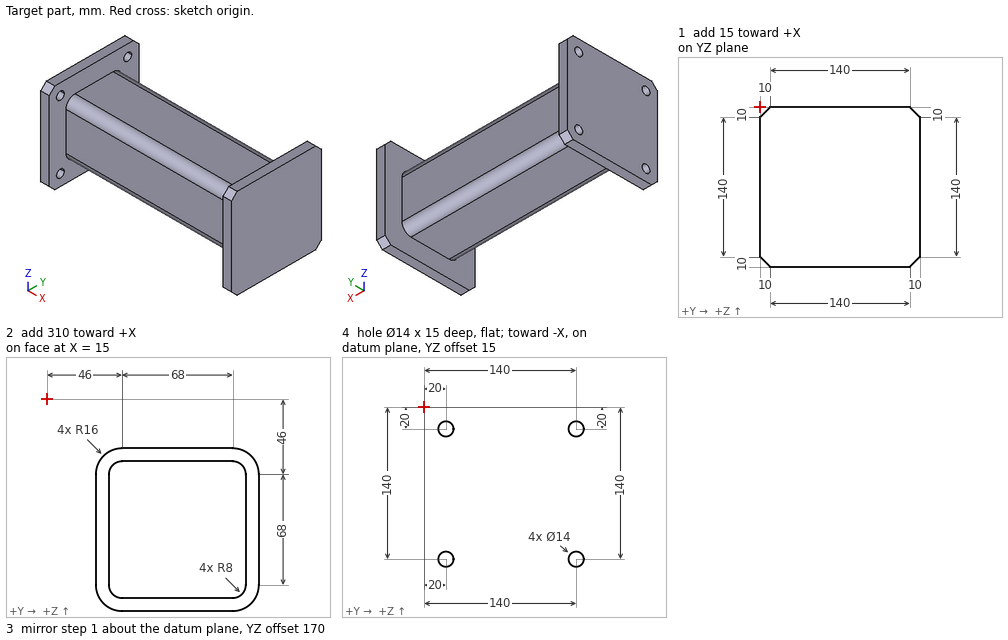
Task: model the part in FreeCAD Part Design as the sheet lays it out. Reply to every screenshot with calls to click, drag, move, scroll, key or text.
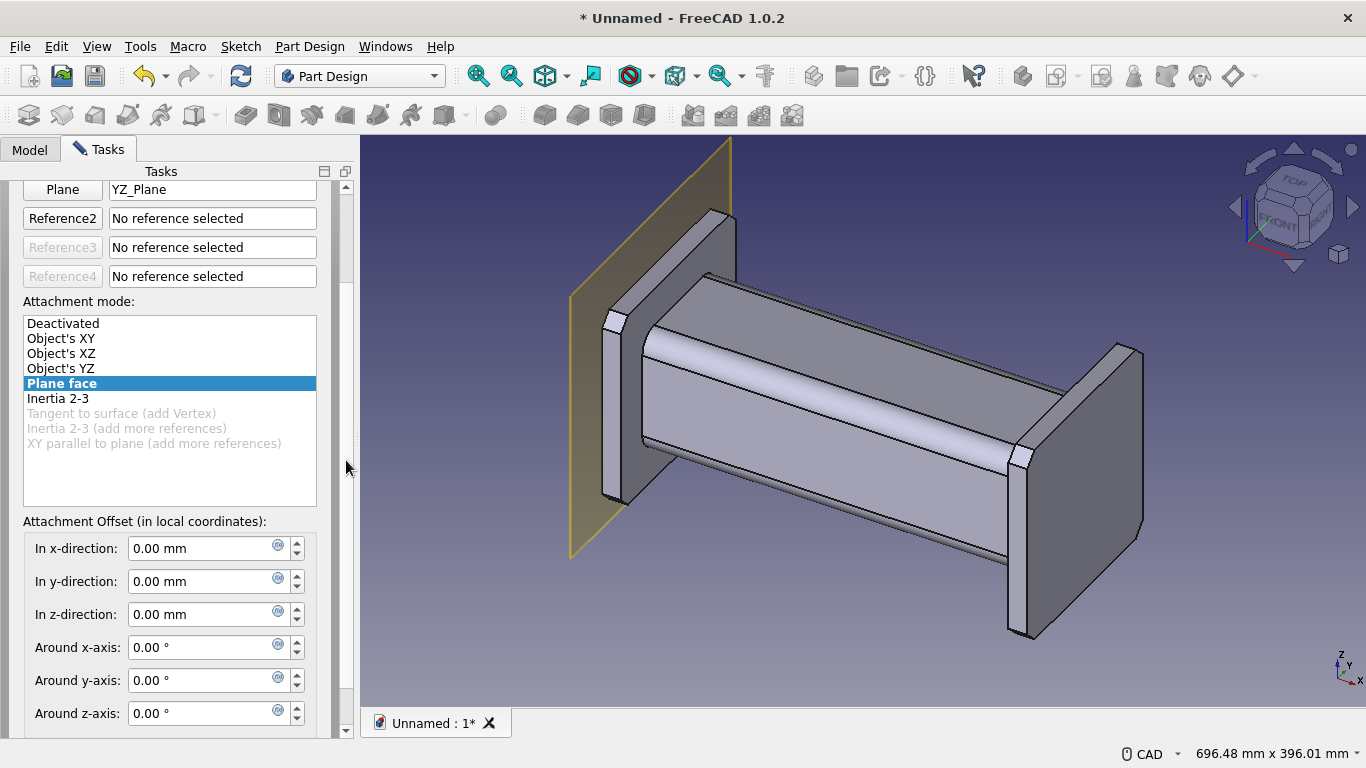
triple_click(210, 614)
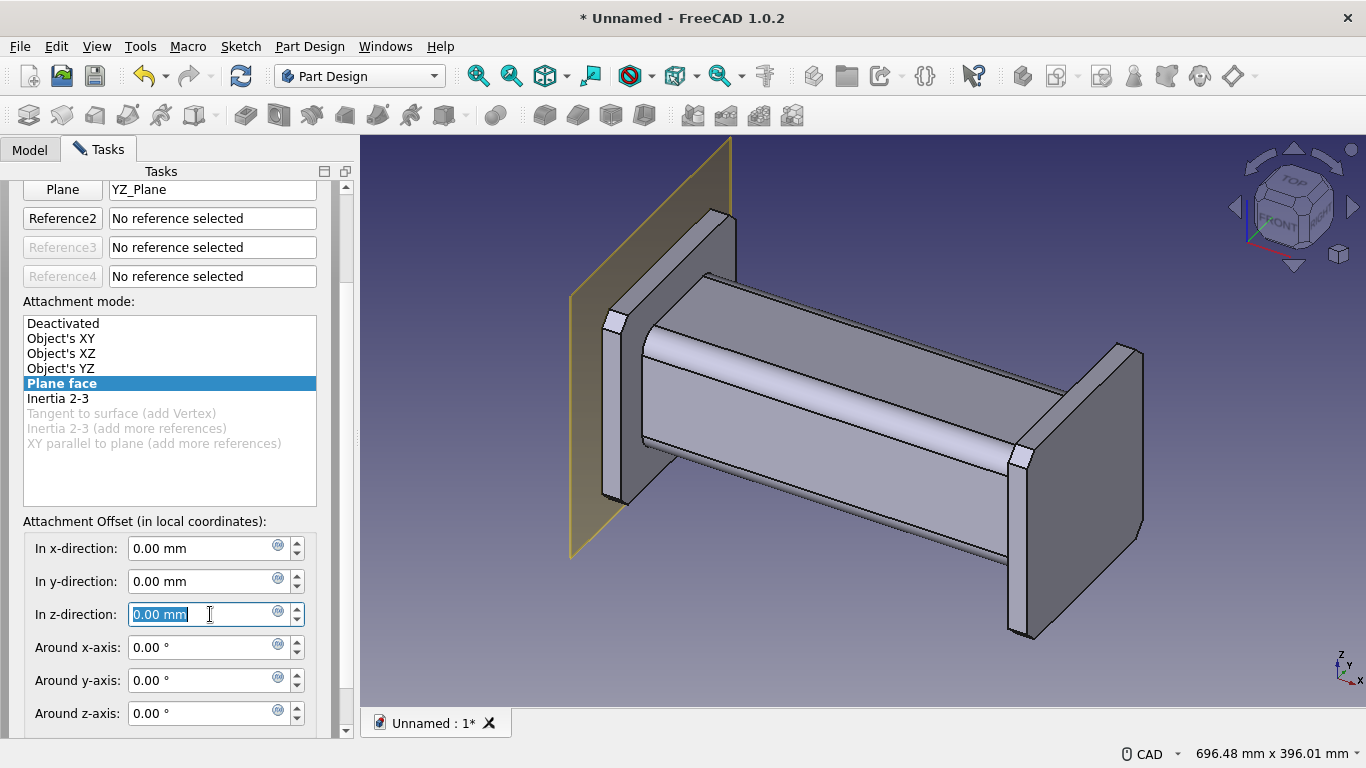
text(15)
key(Tab)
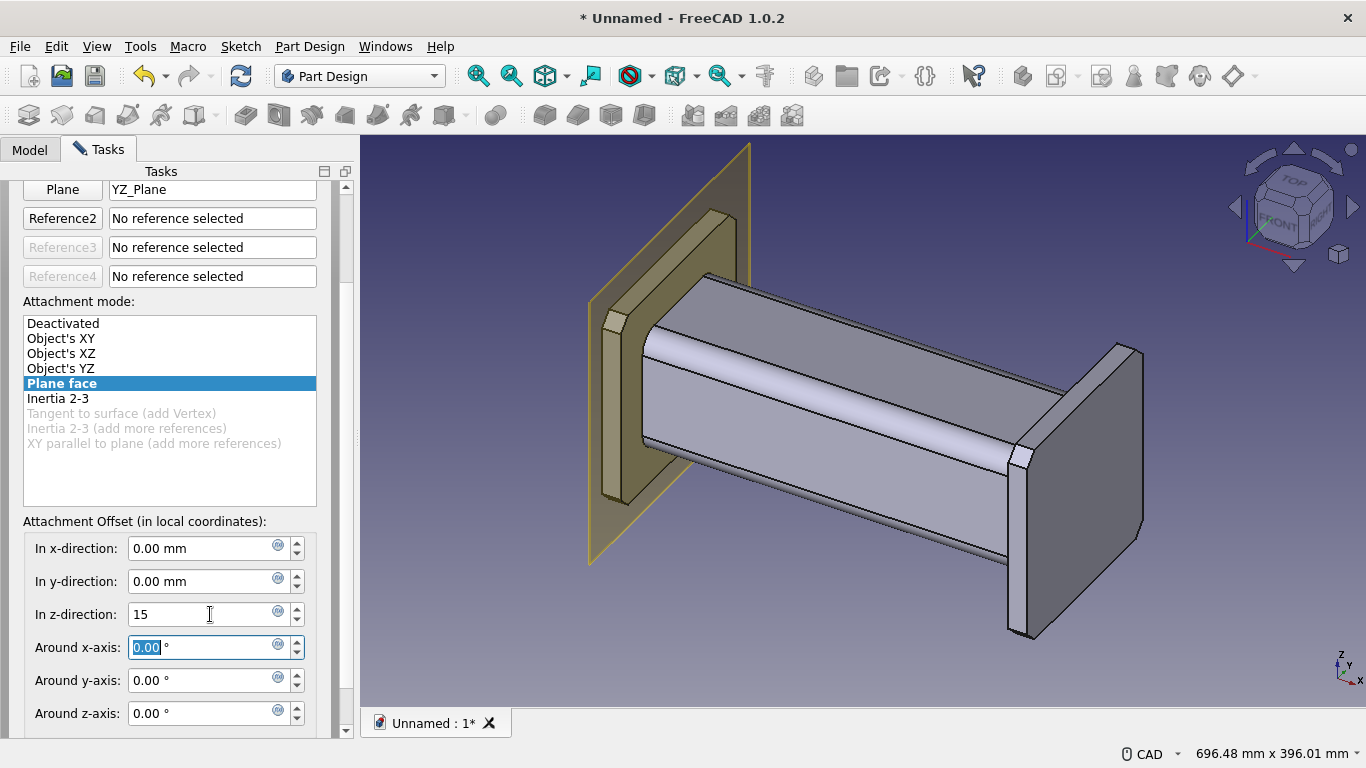
scroll(346, 460, up, 3)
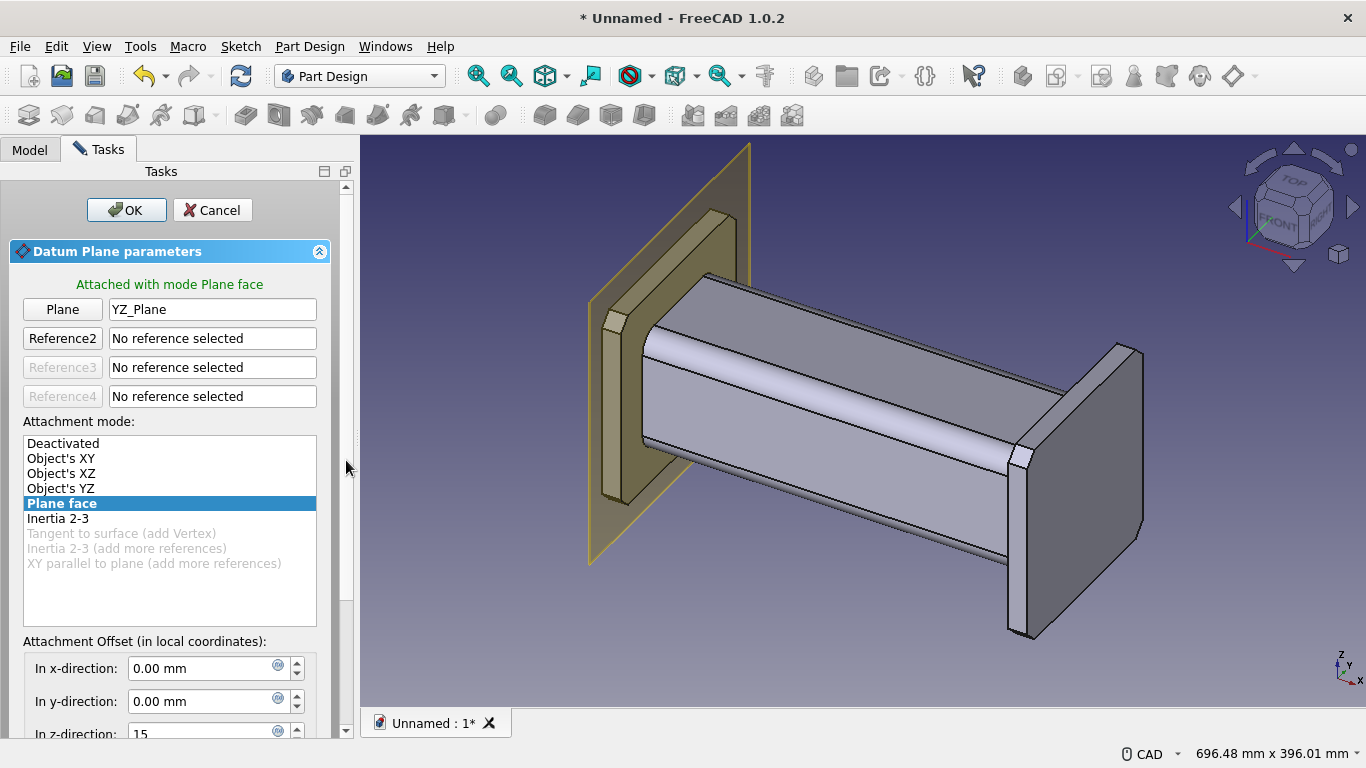
click(127, 210)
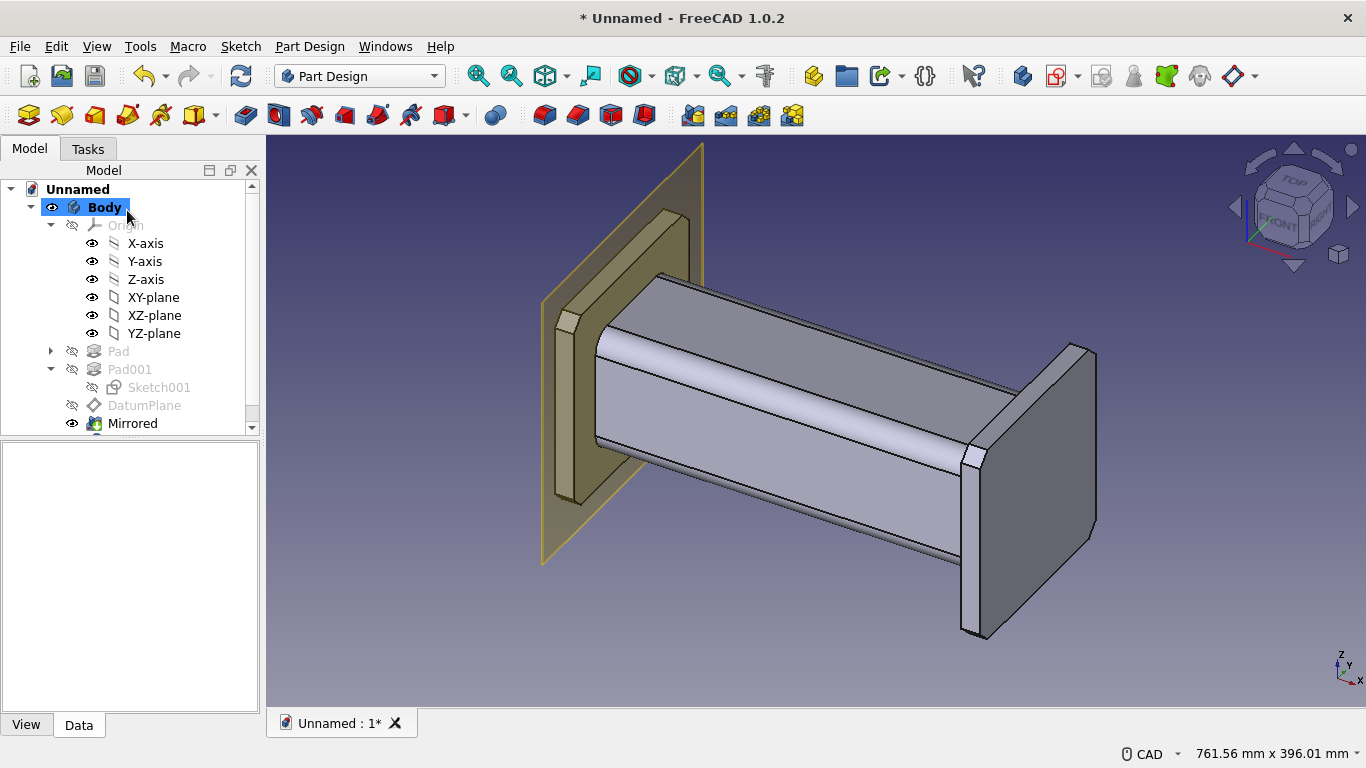
scroll(101, 311, down, 3)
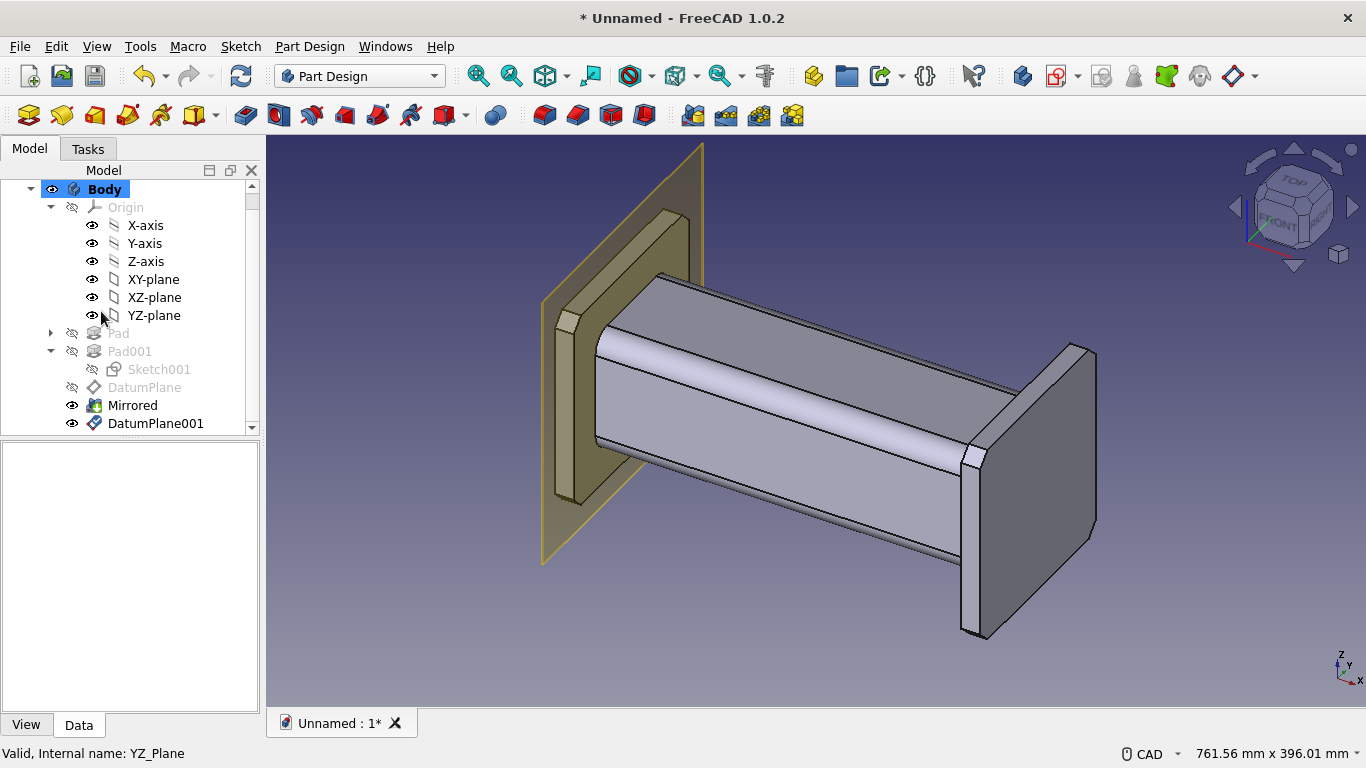
click(117, 423)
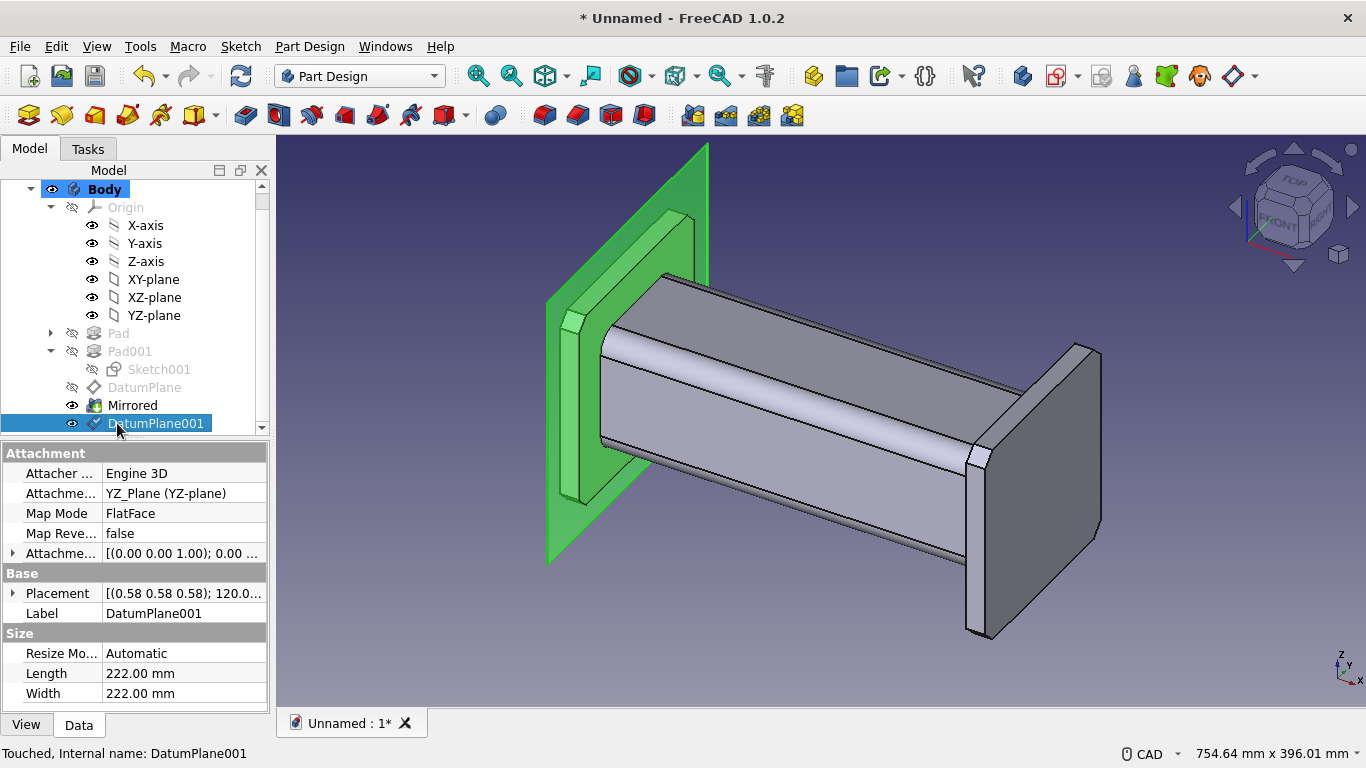
click(1056, 76)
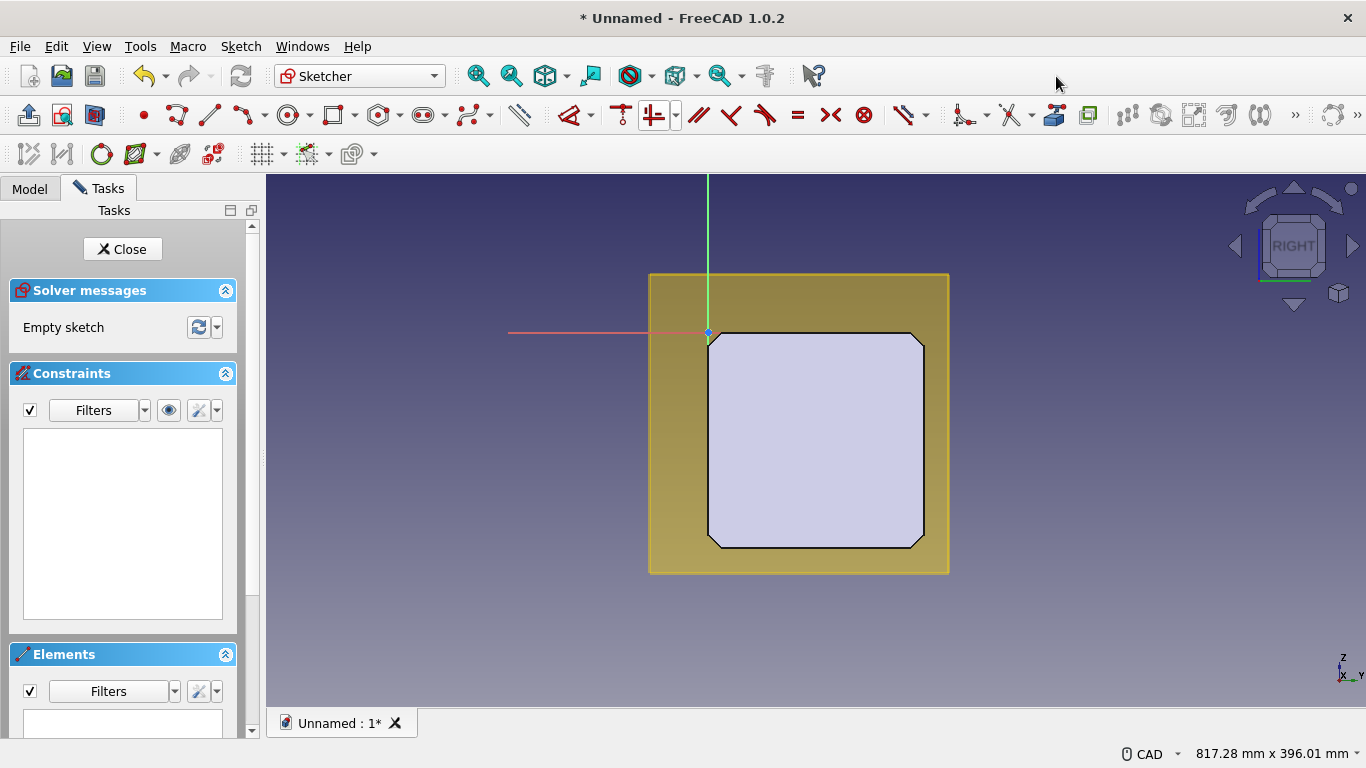
click(95, 116)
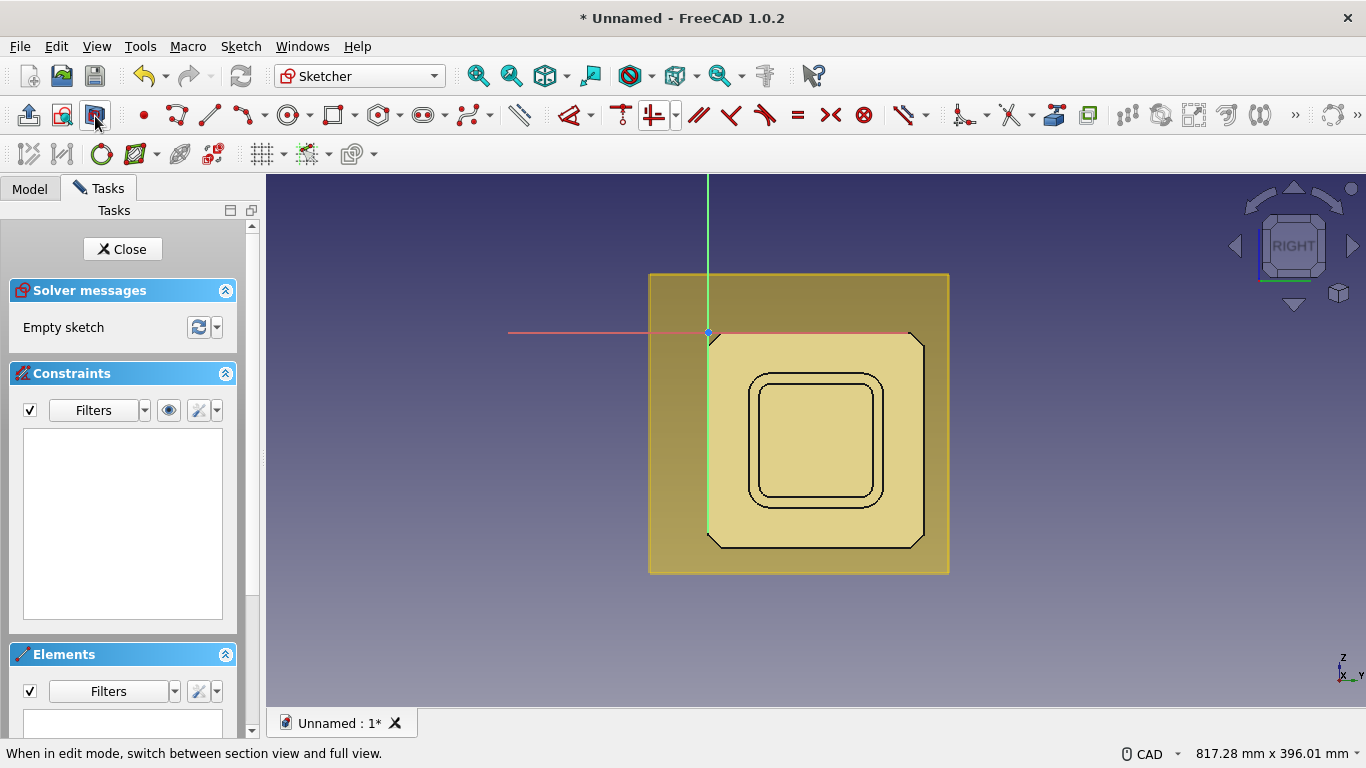
scroll(880, 421, up, 3)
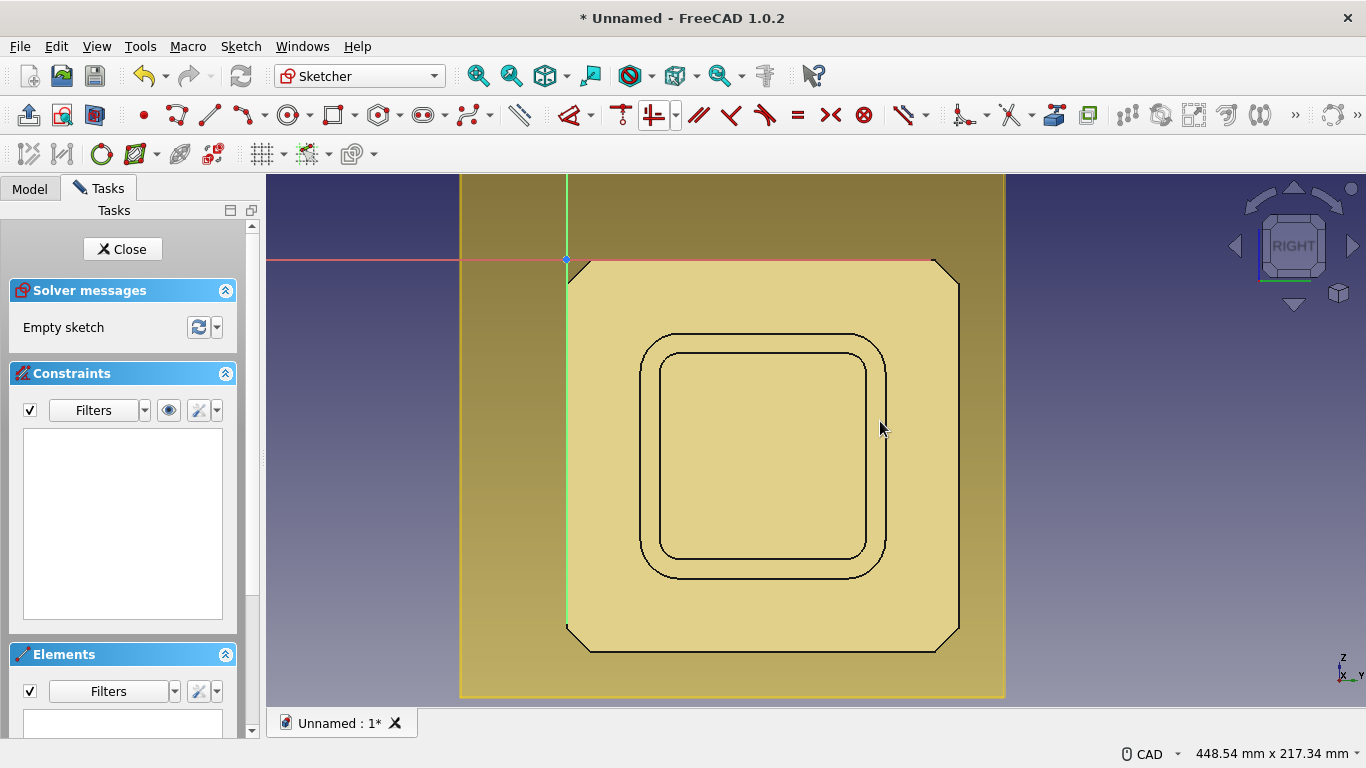
click(288, 116)